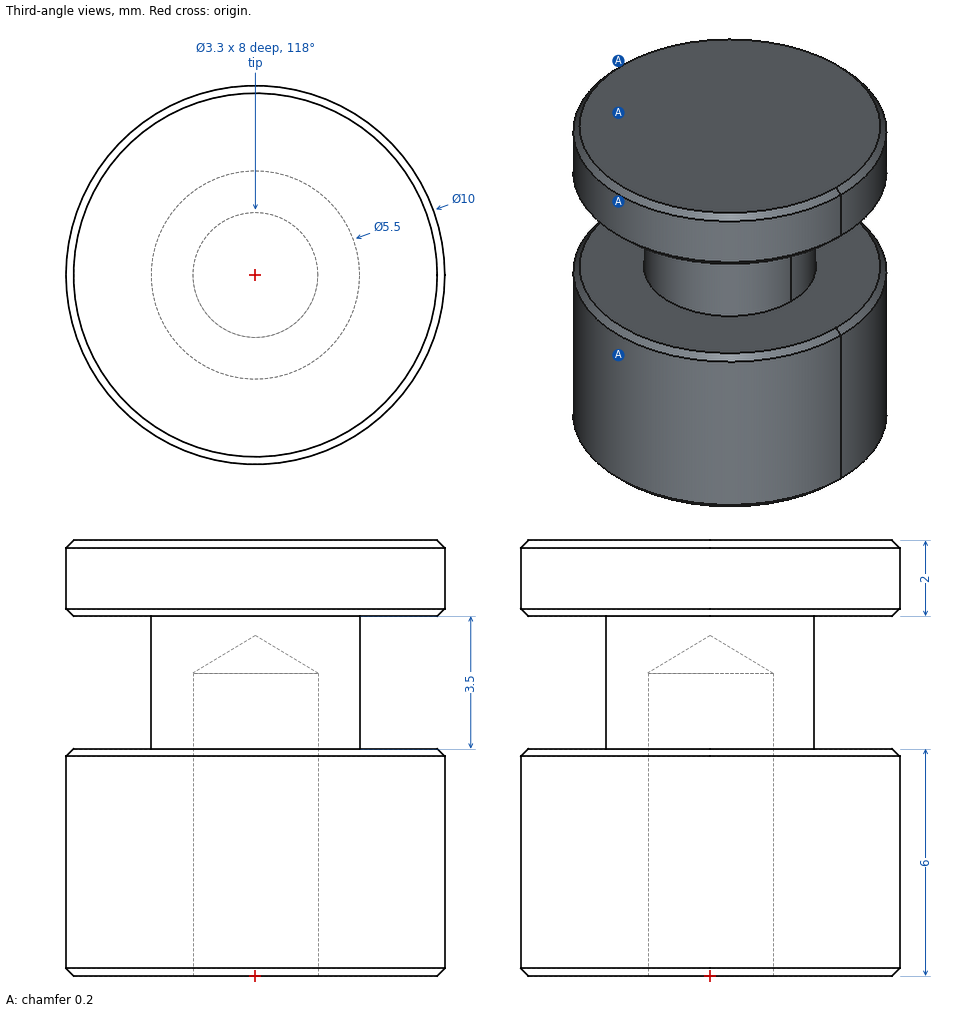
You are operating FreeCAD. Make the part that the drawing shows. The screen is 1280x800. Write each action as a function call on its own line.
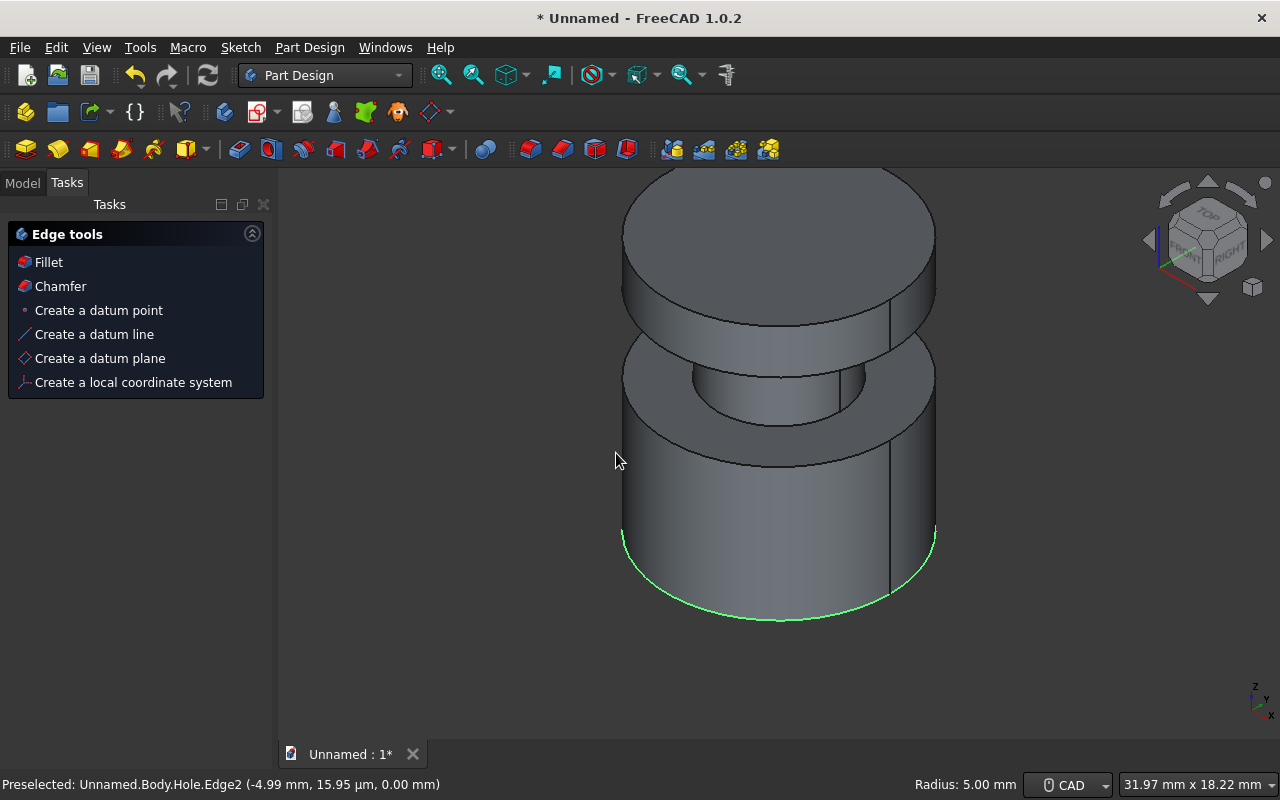
click(442, 76)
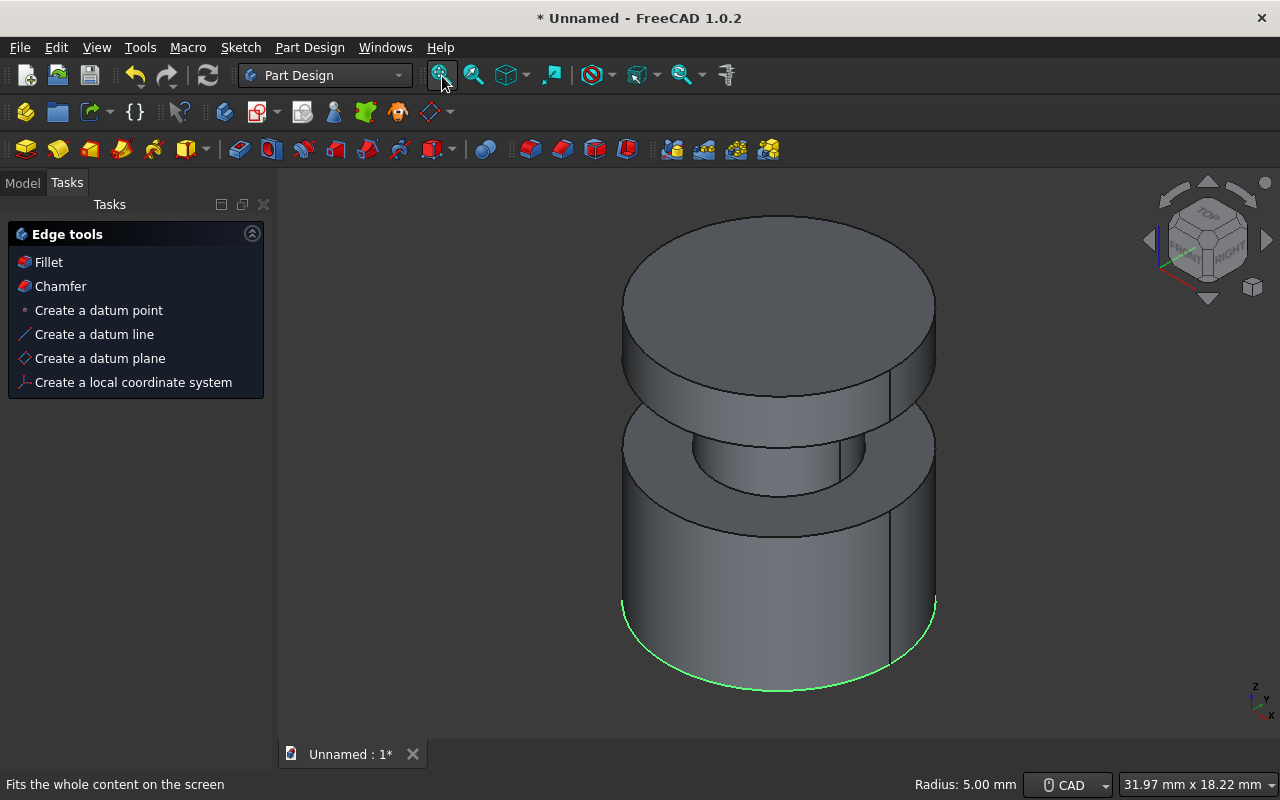
click(639, 487, ctrl)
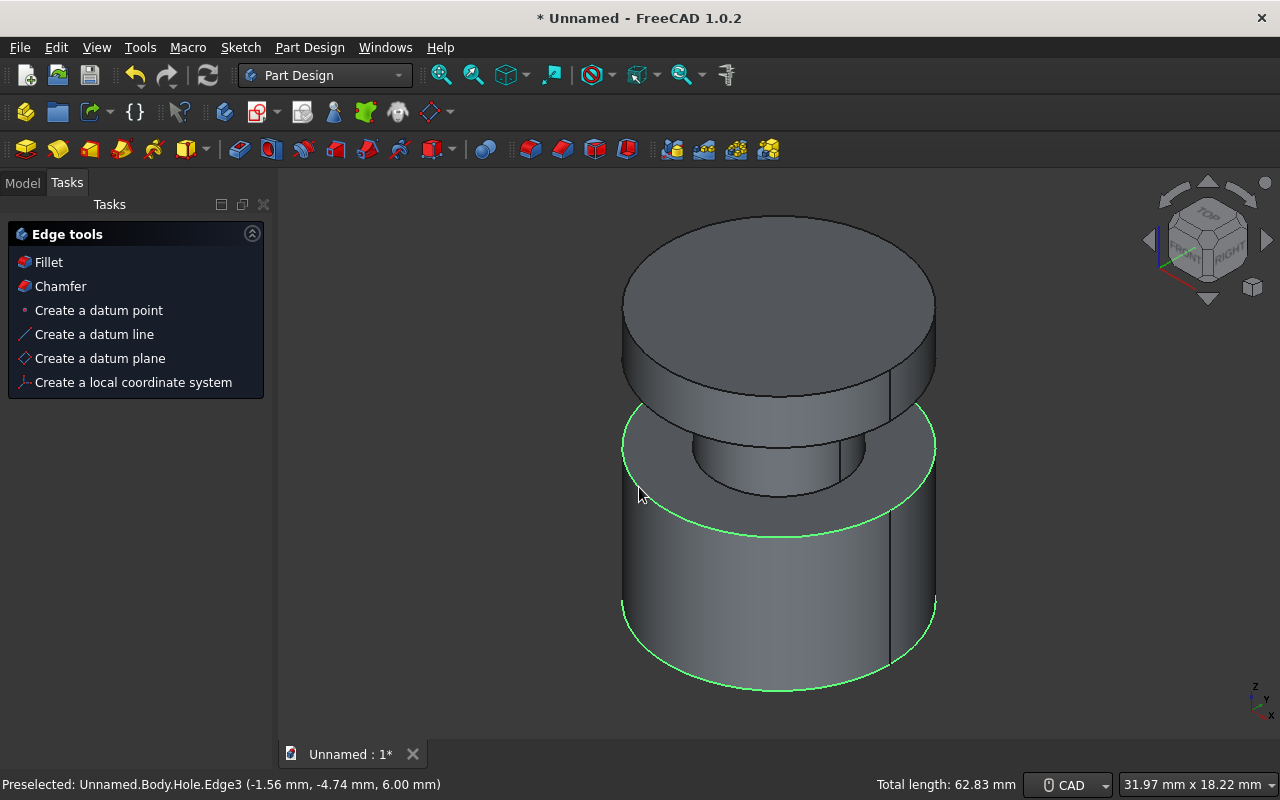
click(639, 346, ctrl)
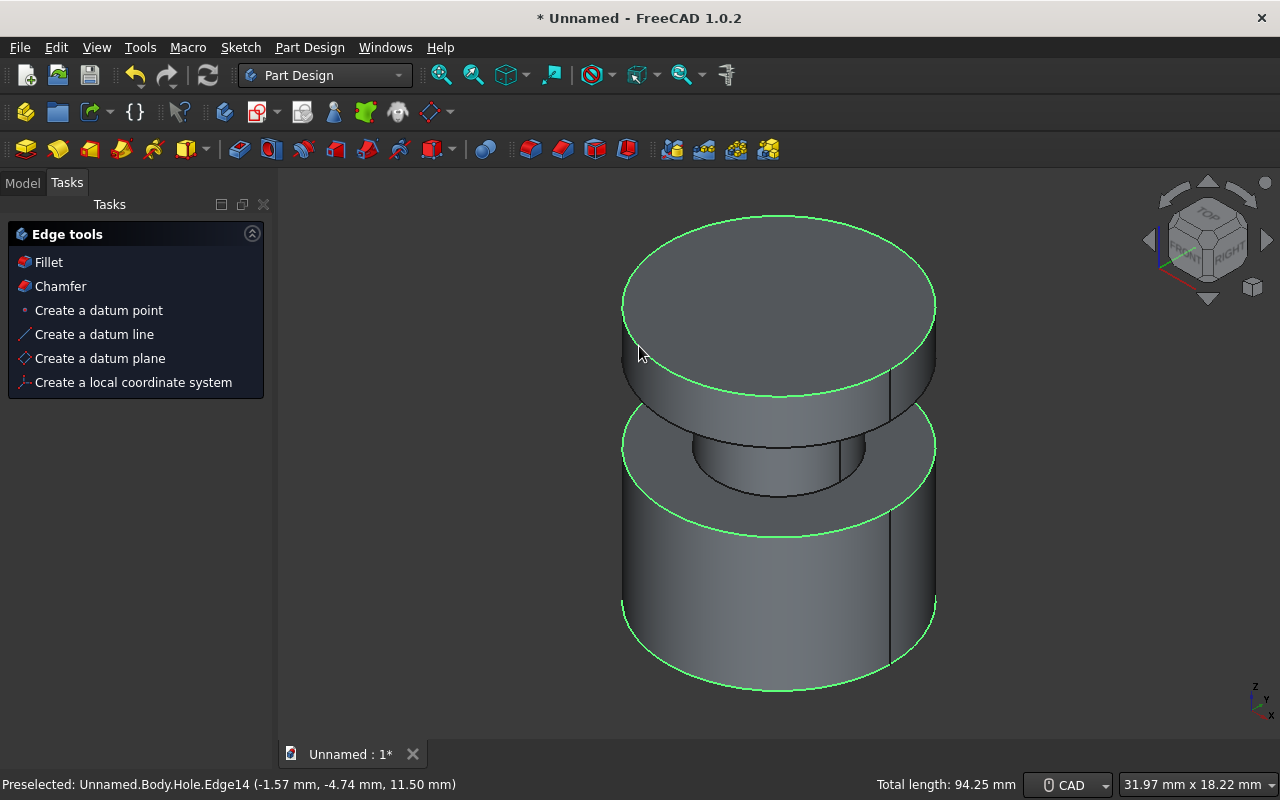
key(2)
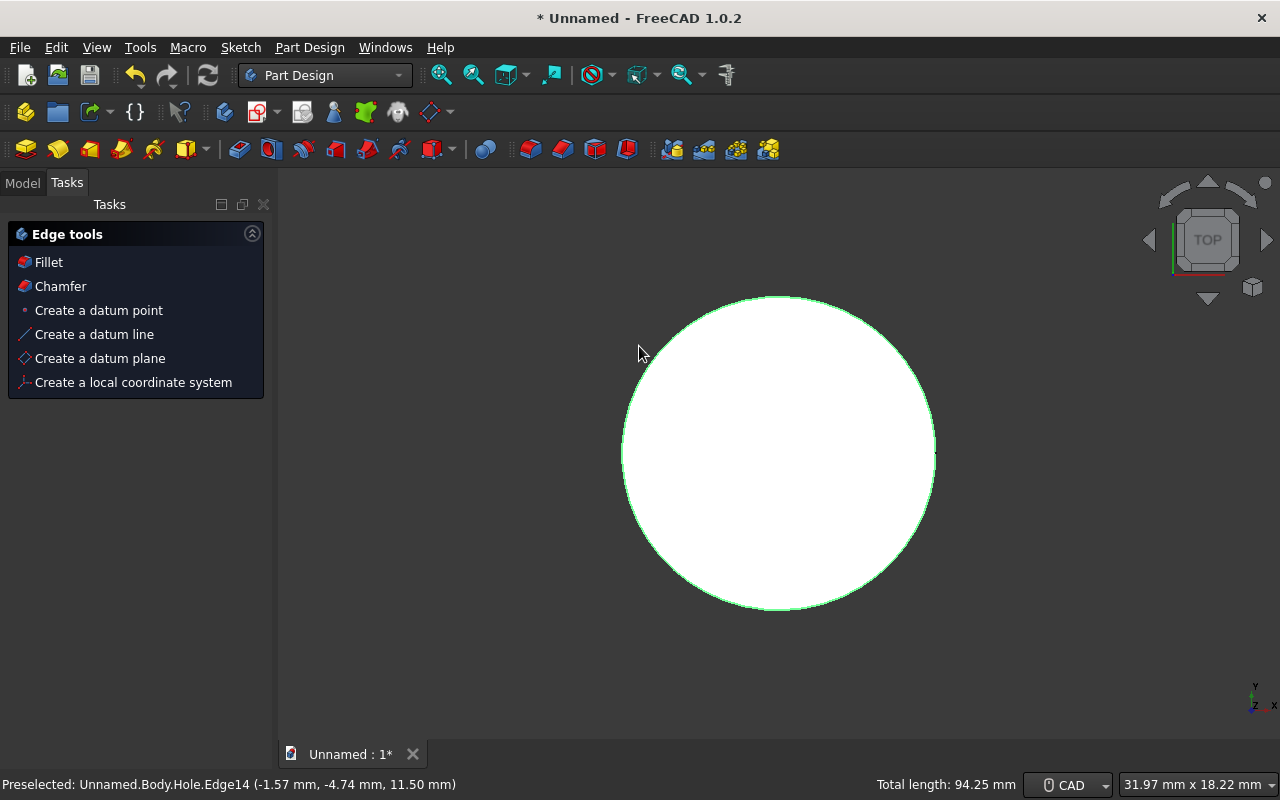
key(1)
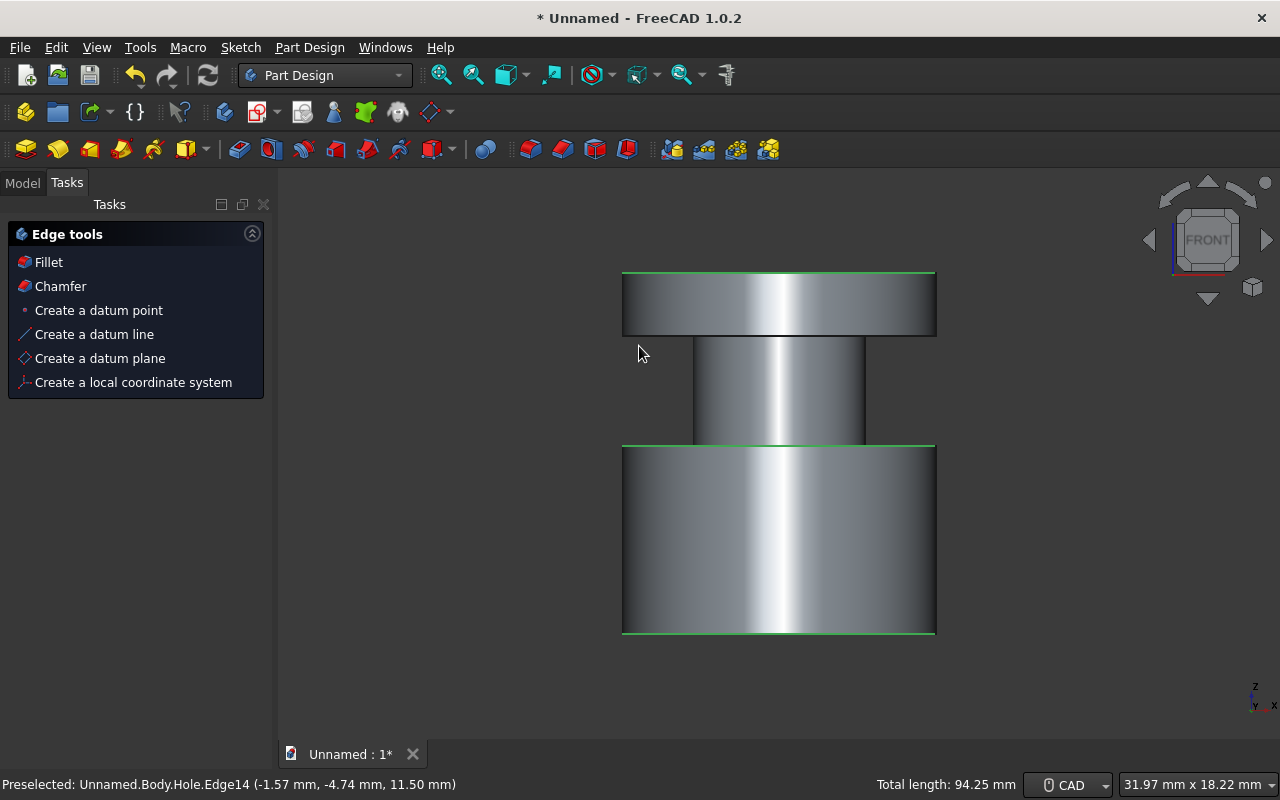
click(652, 335, ctrl)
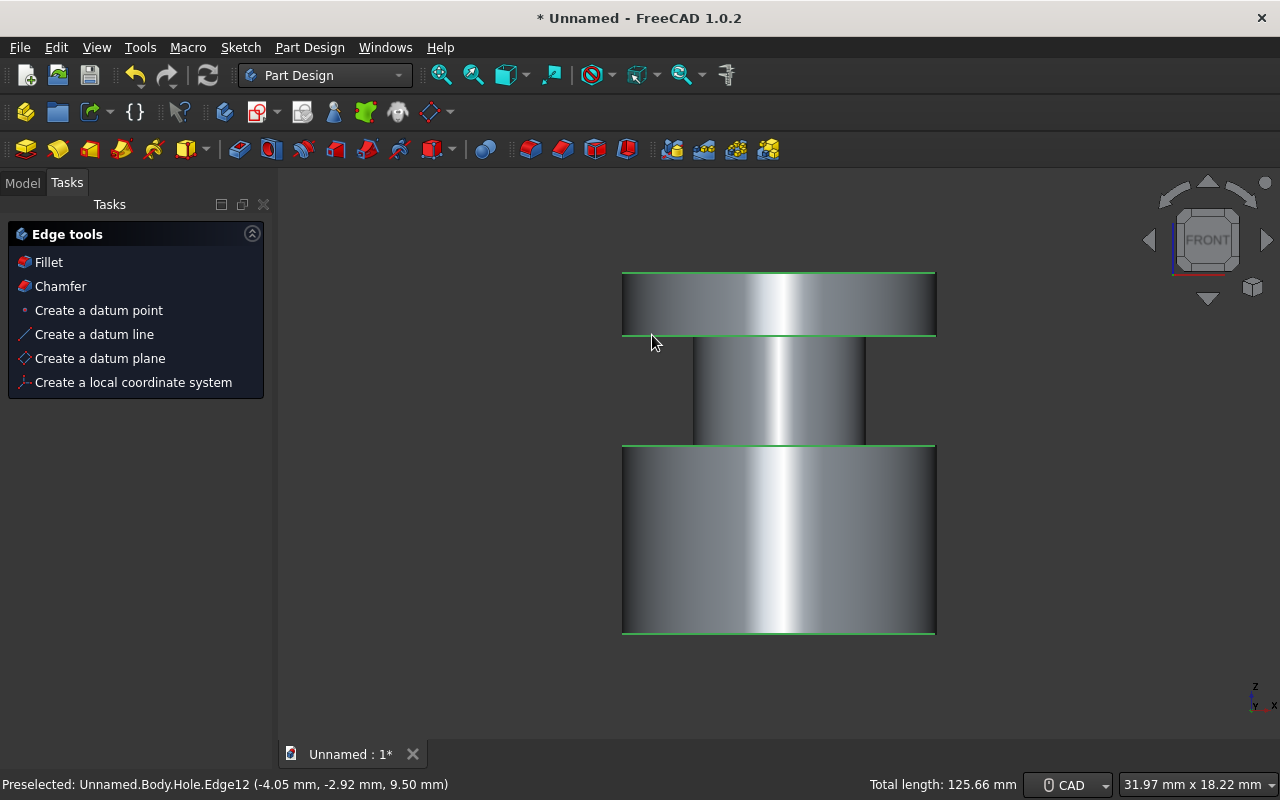
click(564, 150)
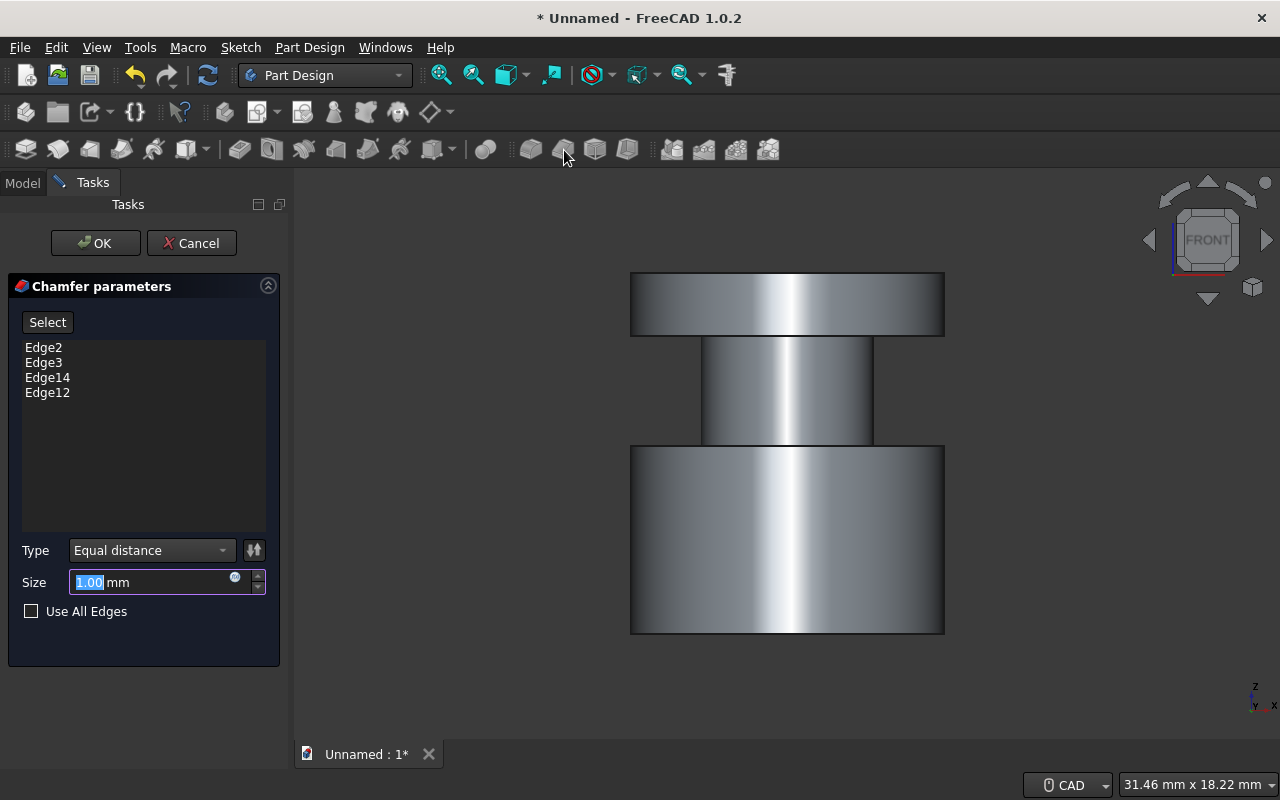
text(0.2)
key(Tab)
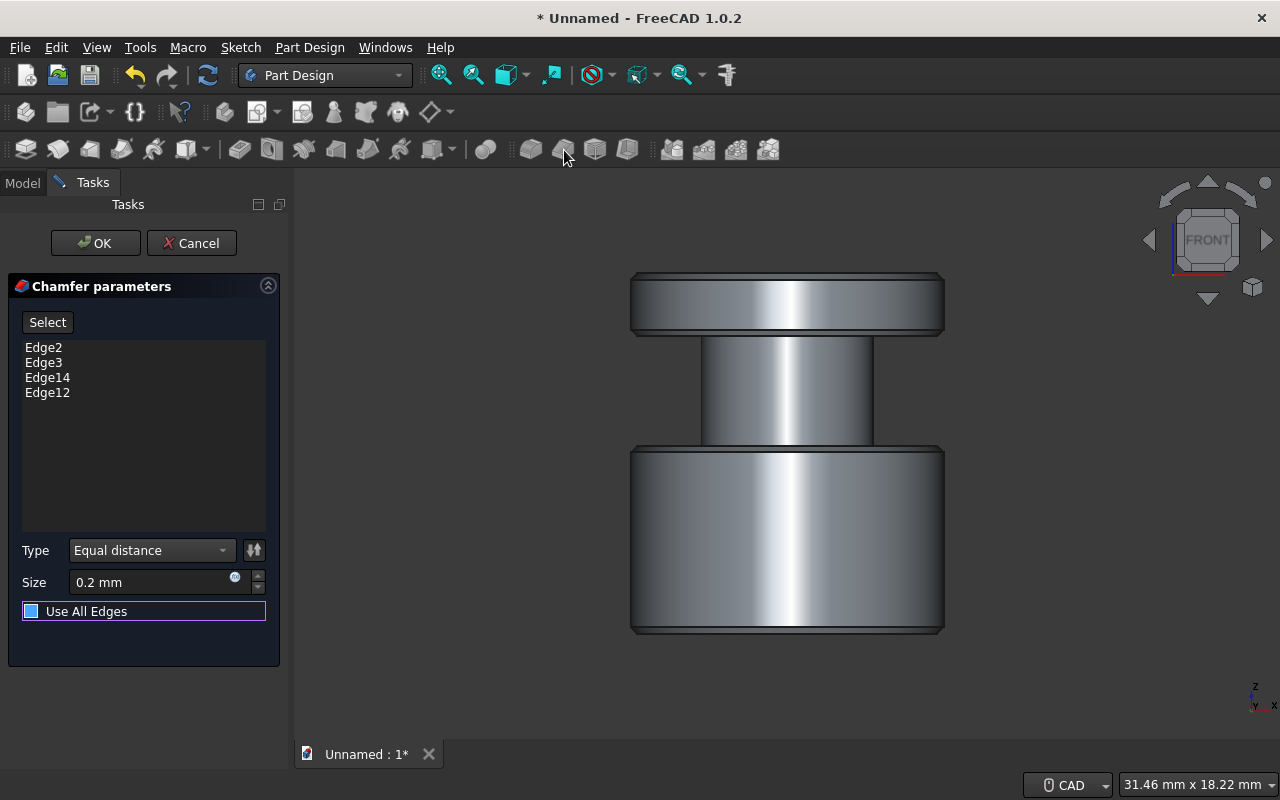
click(96, 243)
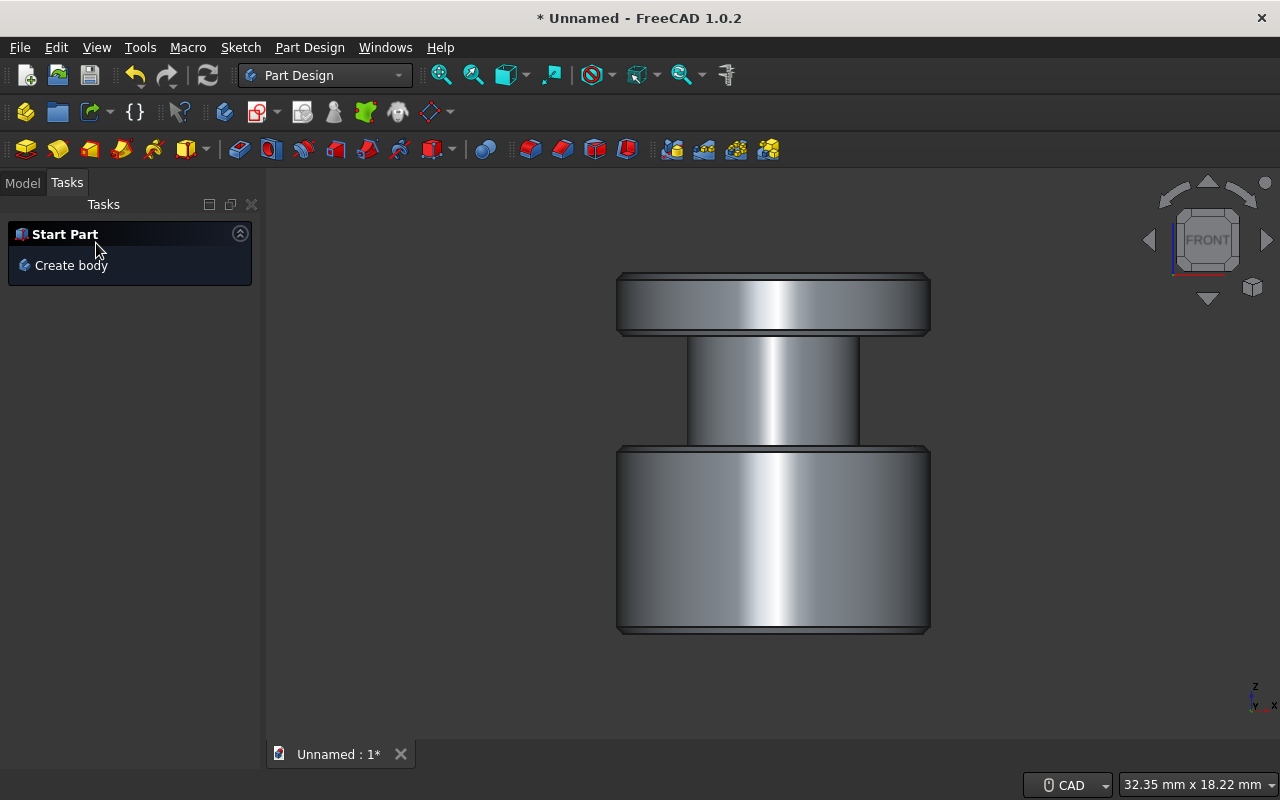
key(0)